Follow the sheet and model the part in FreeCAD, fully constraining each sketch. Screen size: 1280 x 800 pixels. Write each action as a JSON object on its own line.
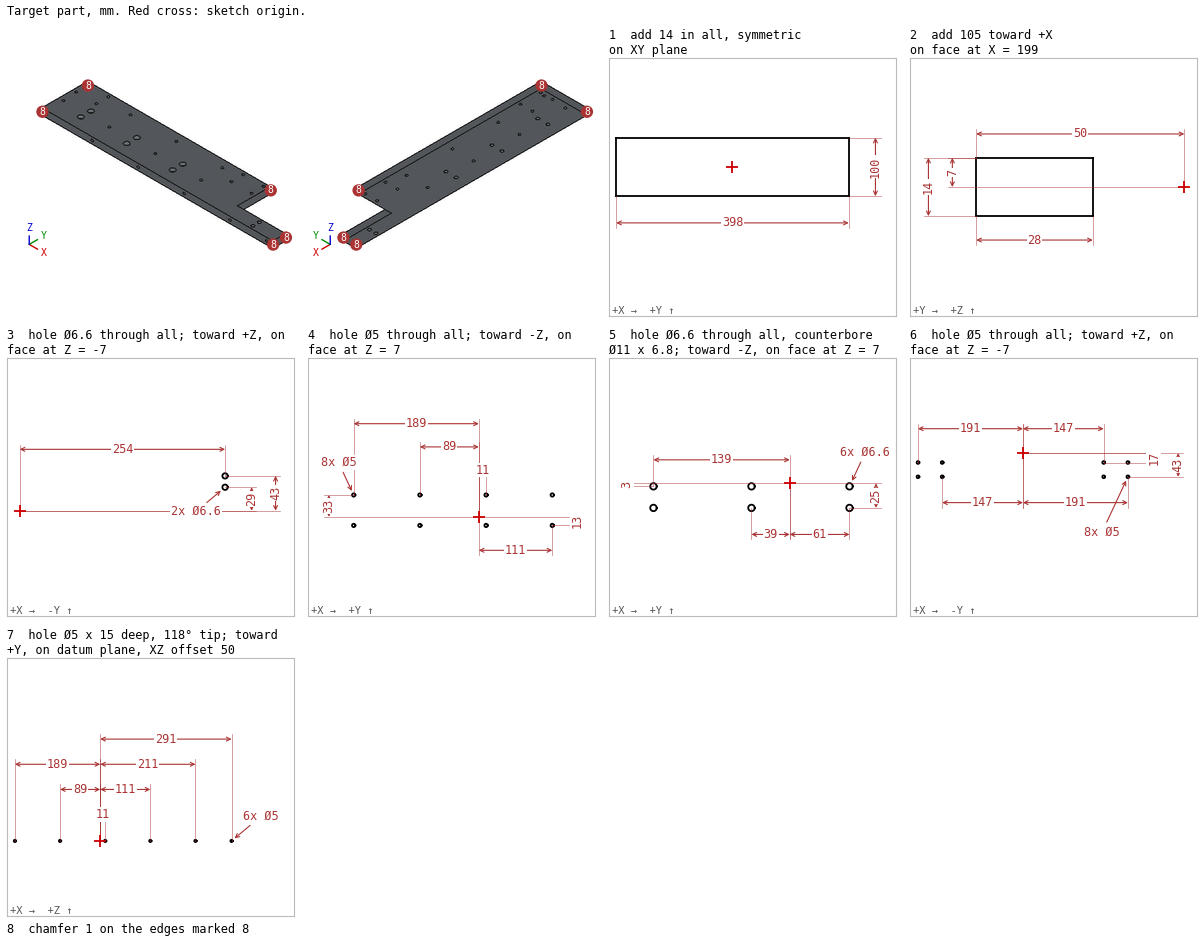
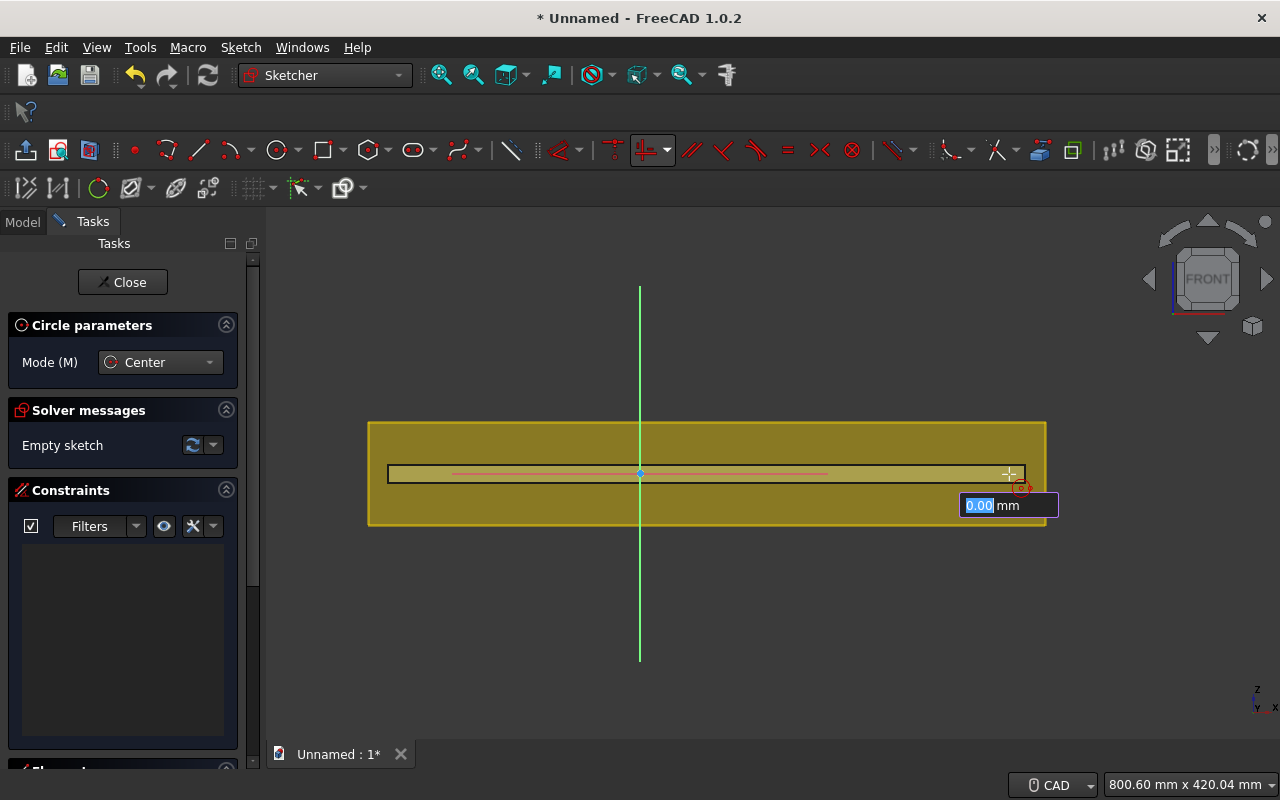
{"action": "scroll", "coordinate": [1008, 477], "scroll_direction": "up", "scroll_amount": 9}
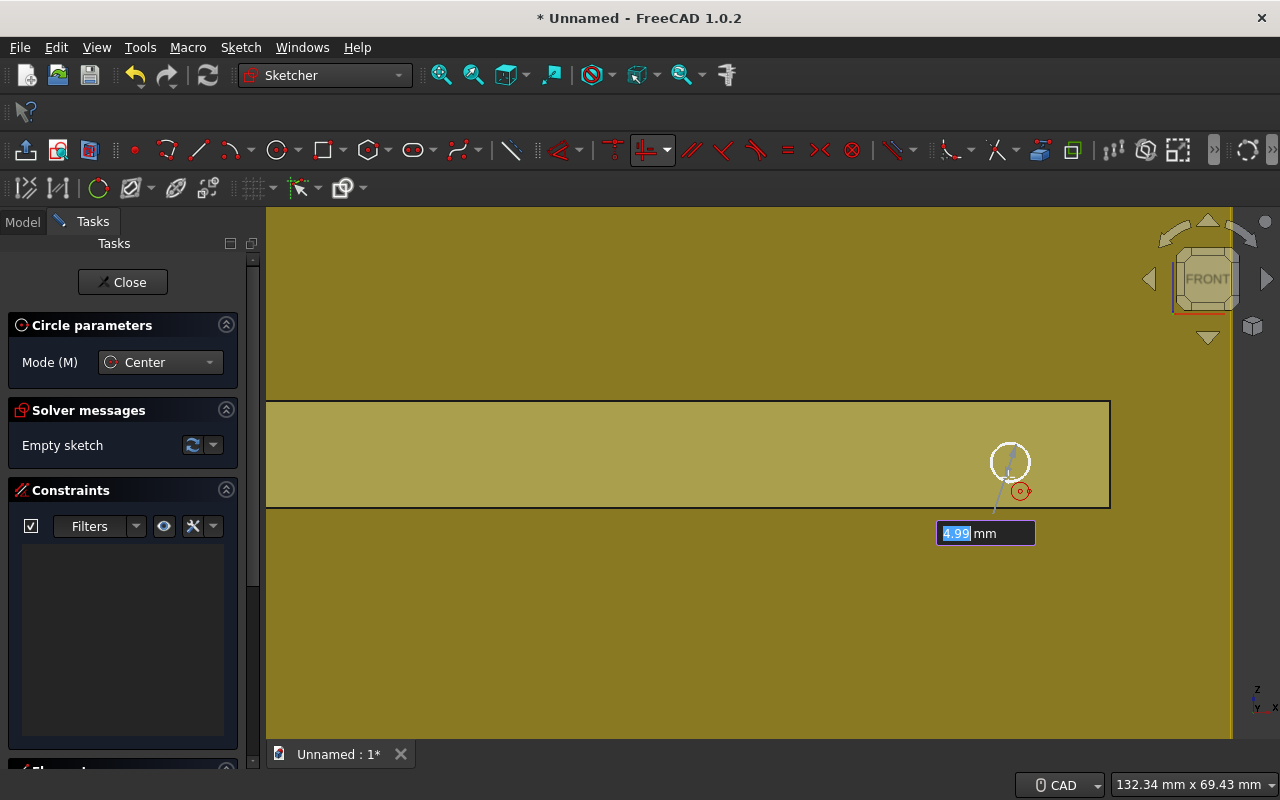
{"action": "left_click", "coordinate": [1004, 473]}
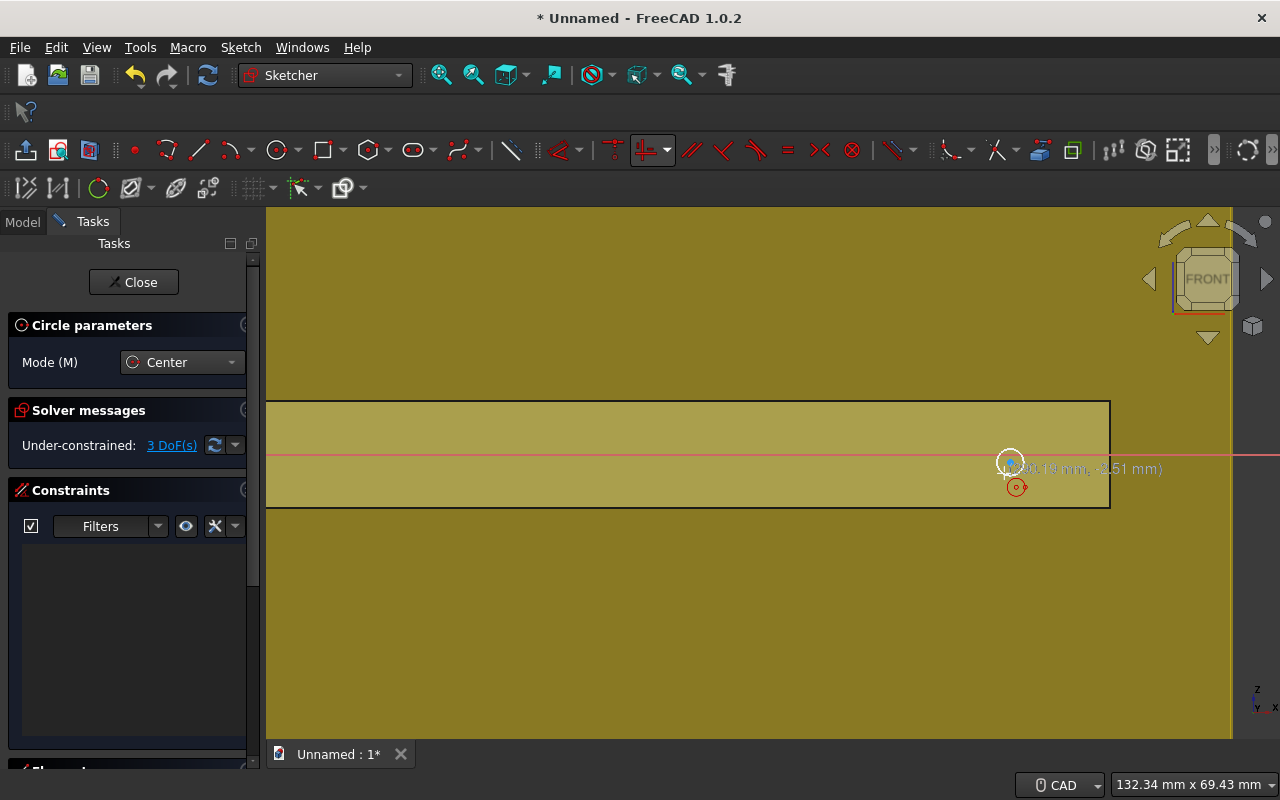
{"action": "scroll", "coordinate": [1008, 477], "scroll_direction": "down", "scroll_amount": 9}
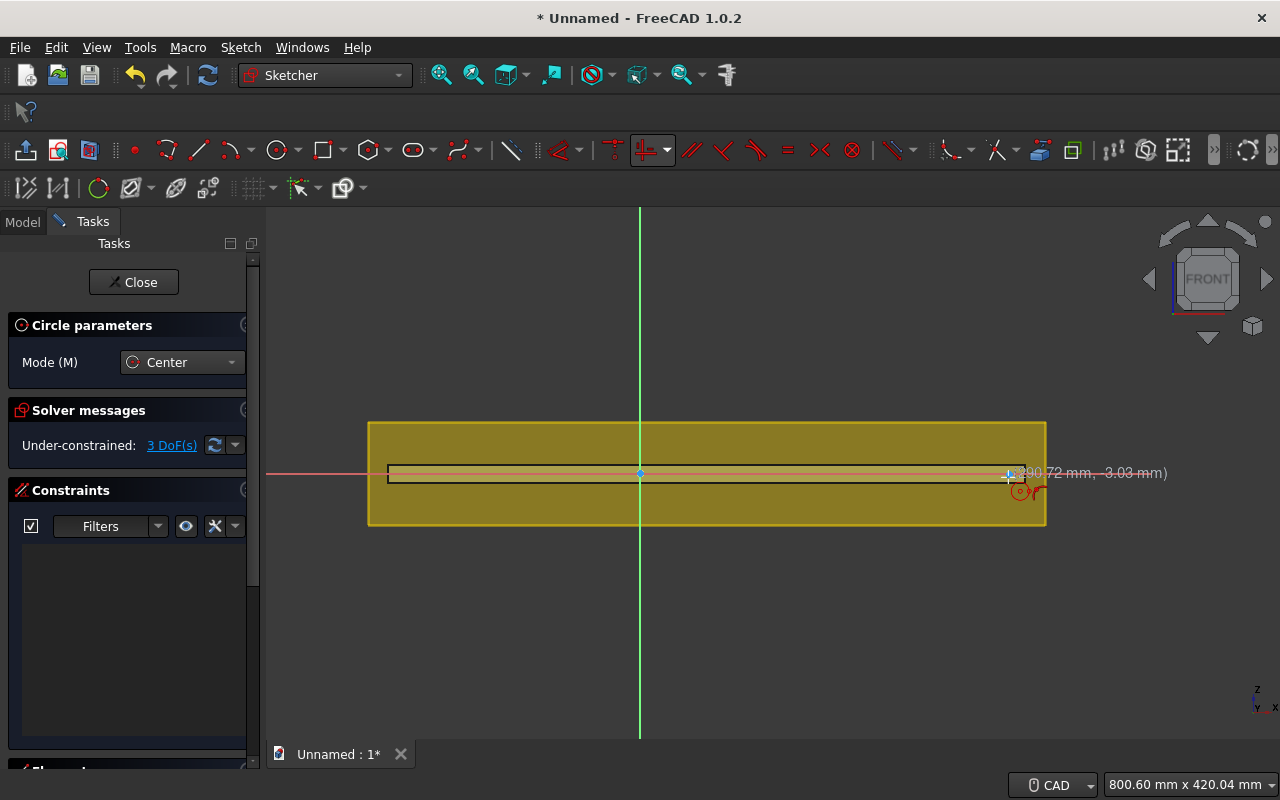
{"action": "scroll", "coordinate": [401, 474], "scroll_direction": "up", "scroll_amount": 10}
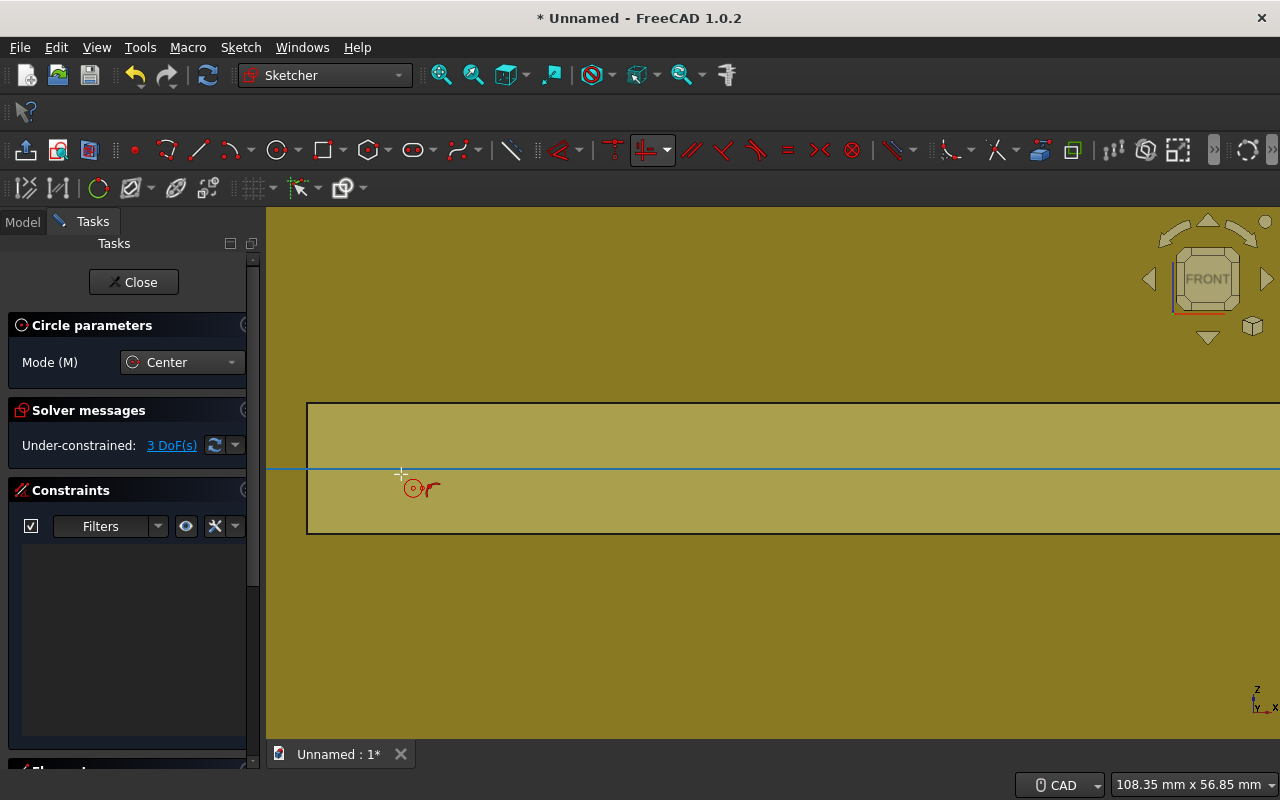
{"action": "scroll", "coordinate": [401, 474], "scroll_direction": "down", "scroll_amount": 10}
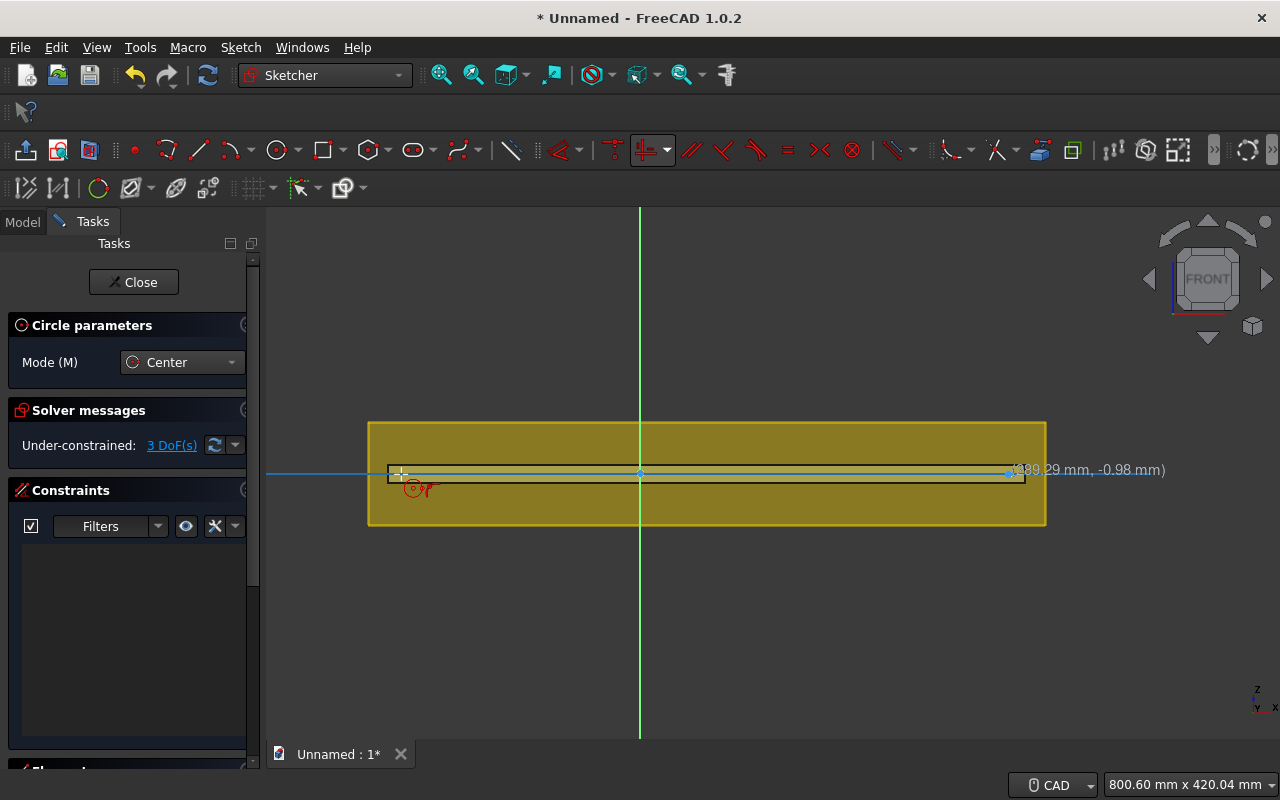
{"action": "left_click", "coordinate": [401, 474]}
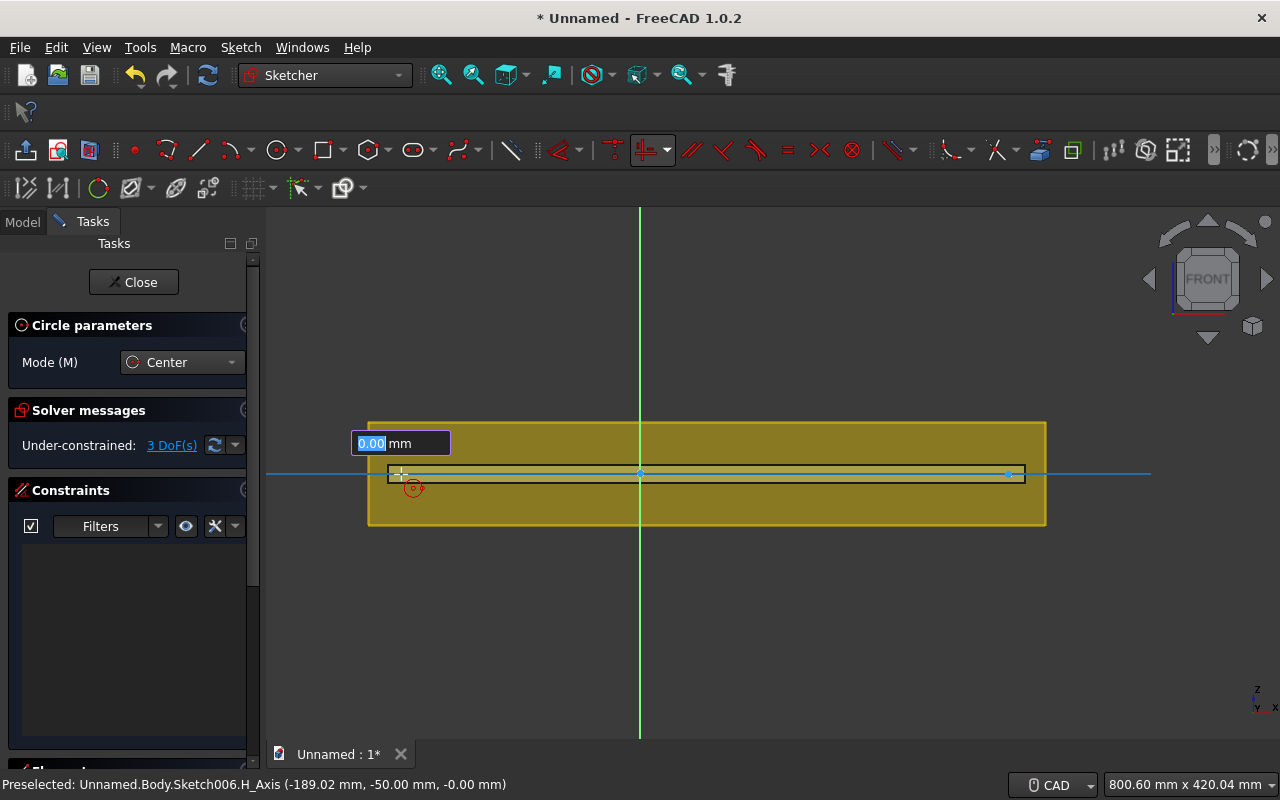
{"action": "scroll", "coordinate": [400, 477], "scroll_direction": "up", "scroll_amount": 9}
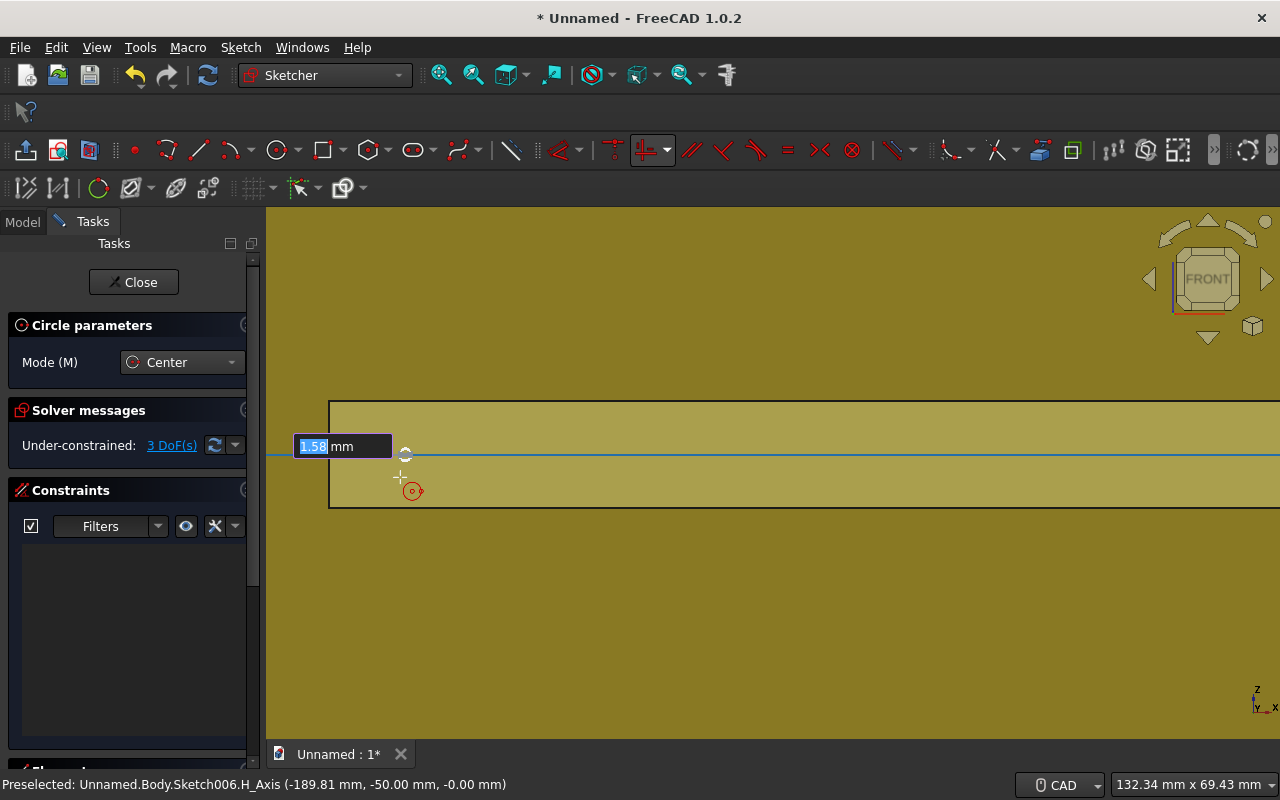
{"action": "left_click", "coordinate": [399, 473]}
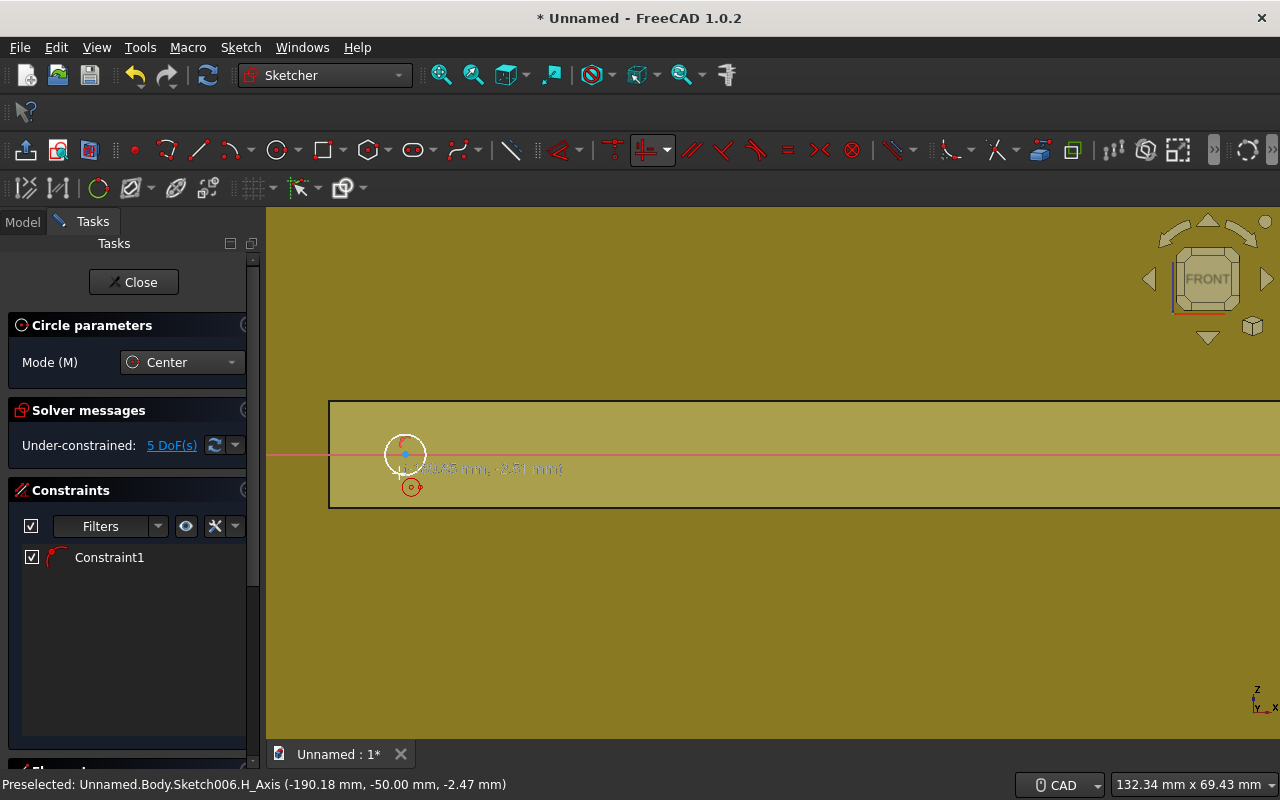
{"action": "scroll", "coordinate": [400, 477], "scroll_direction": "down", "scroll_amount": 9}